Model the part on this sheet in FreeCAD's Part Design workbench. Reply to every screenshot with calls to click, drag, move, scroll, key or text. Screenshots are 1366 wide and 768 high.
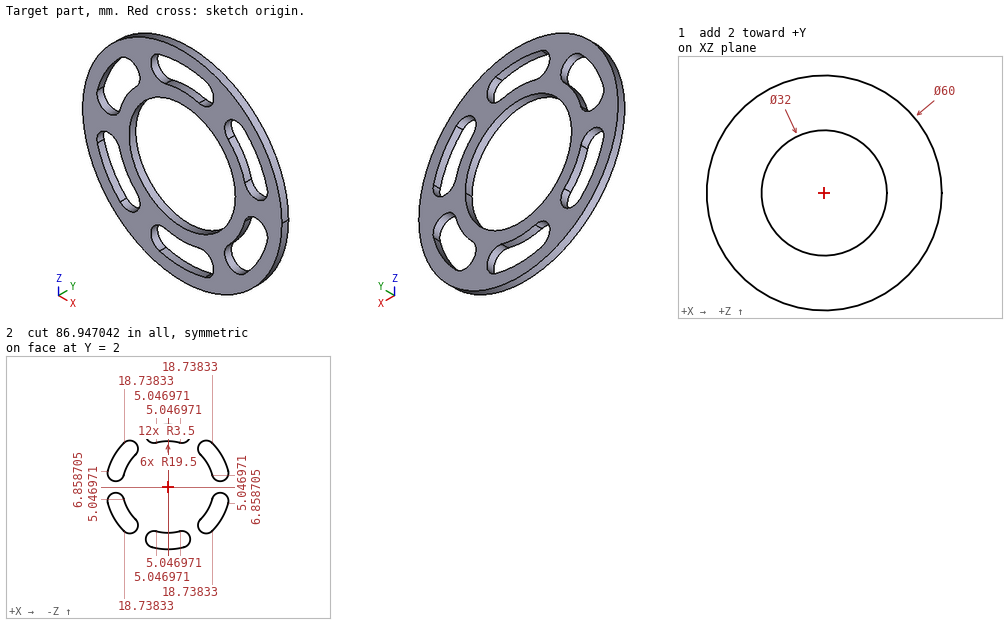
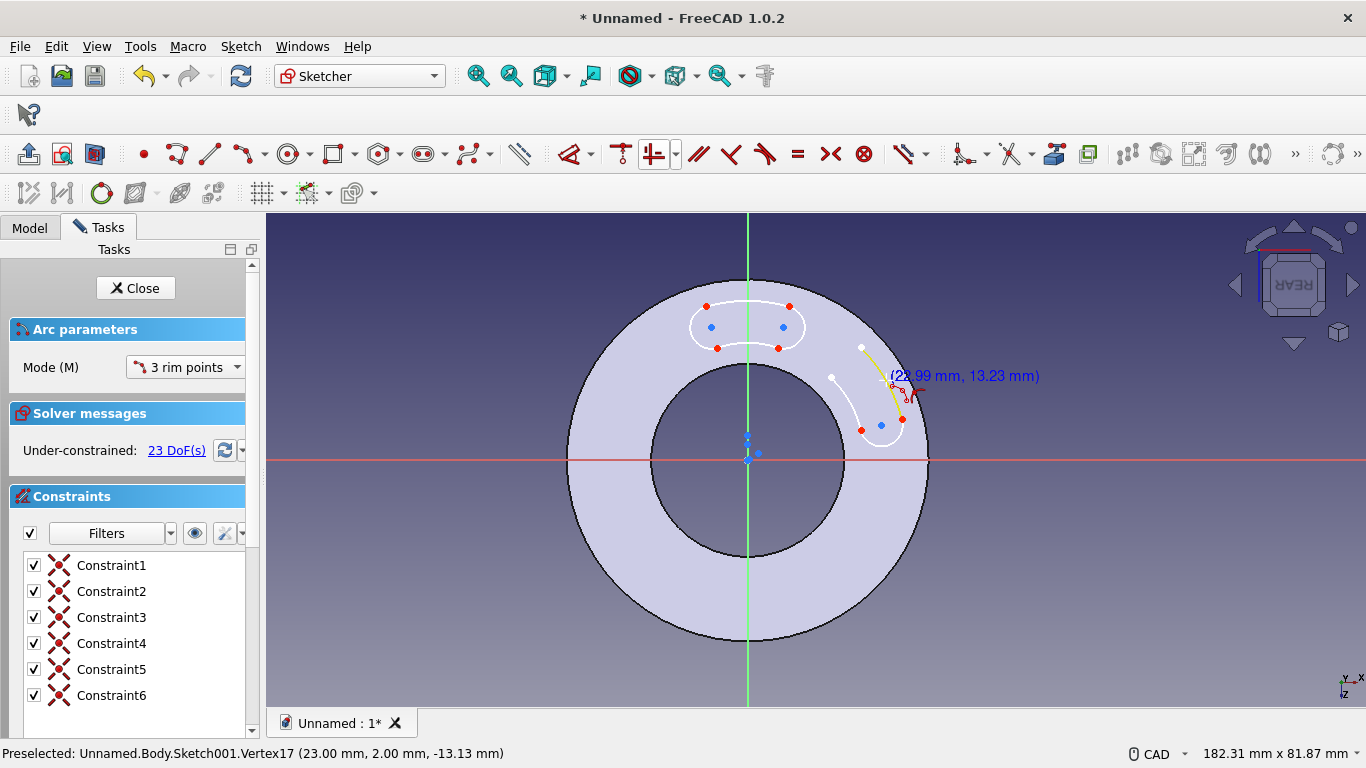
click(861, 348)
click(831, 378)
click(831, 347)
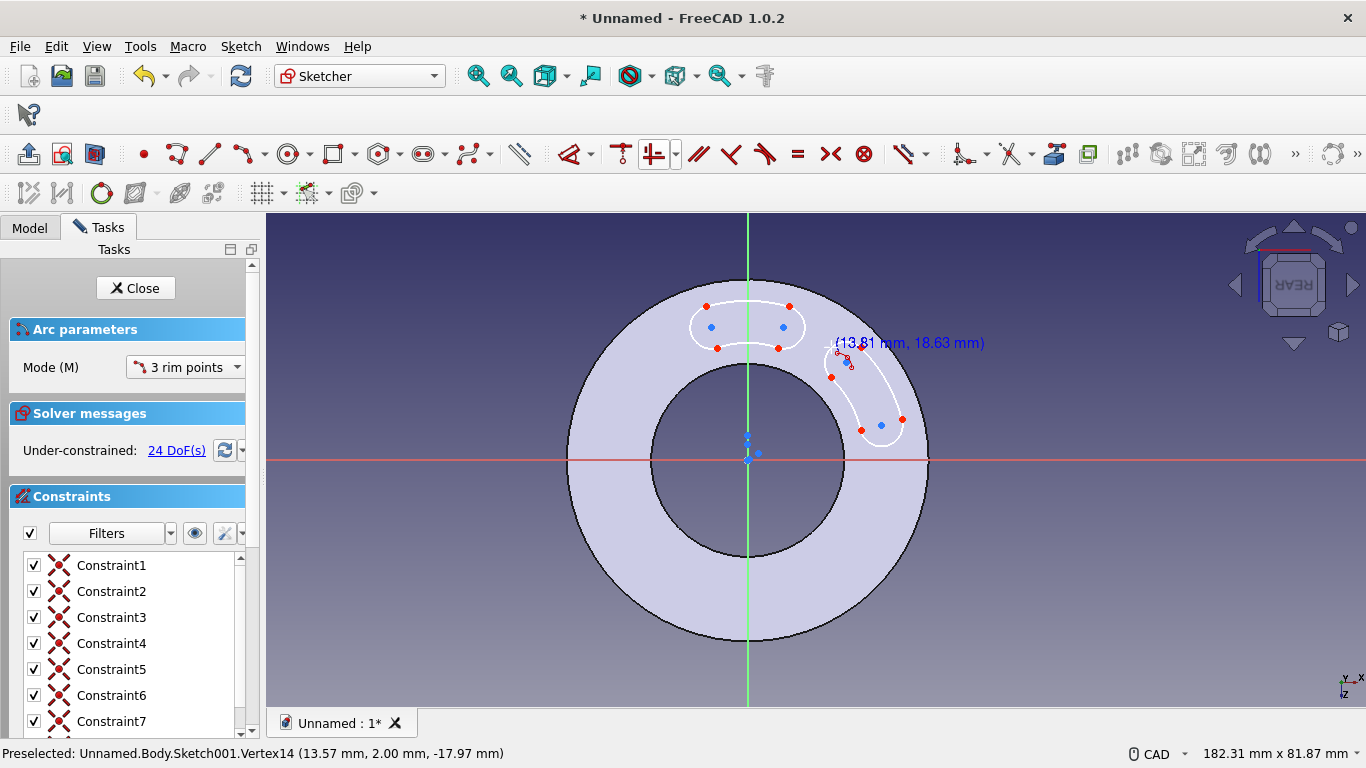
click(831, 544)
click(861, 573)
click(831, 573)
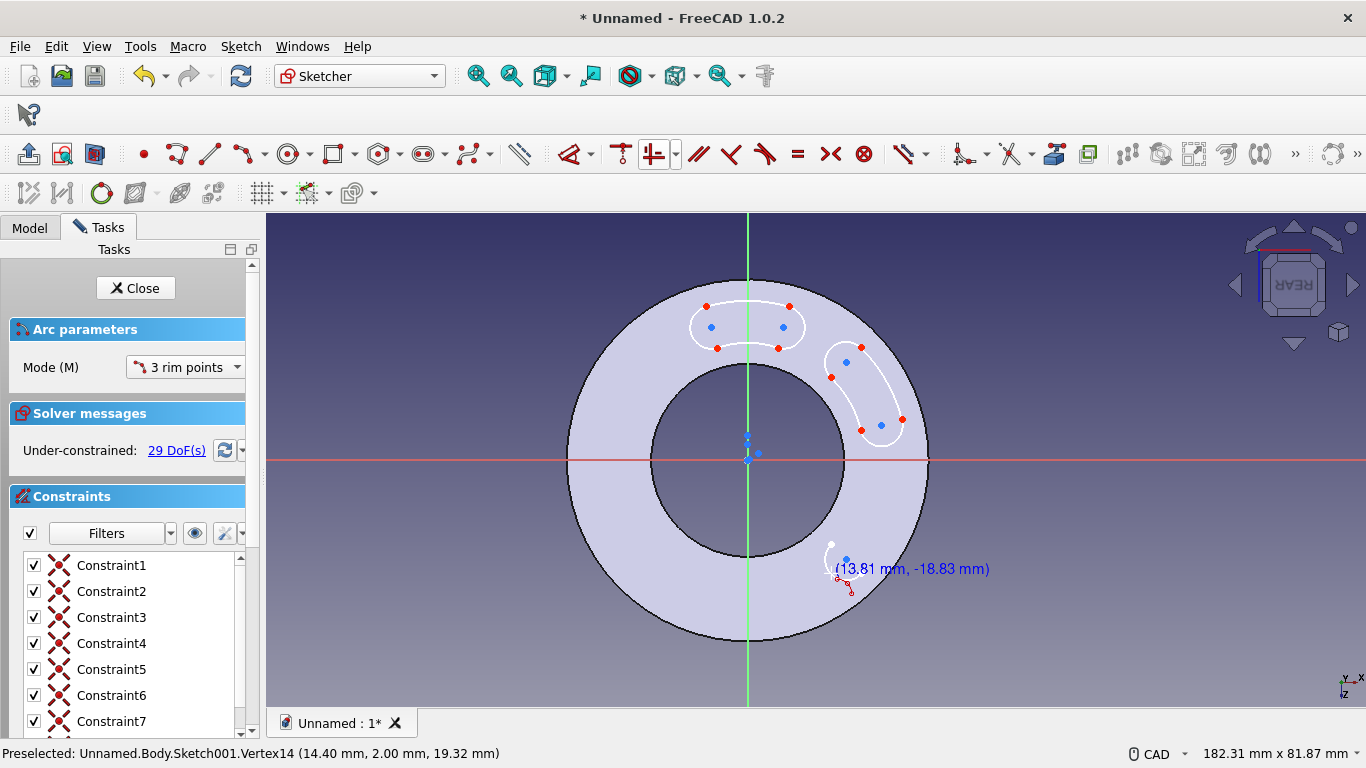
click(861, 574)
click(902, 502)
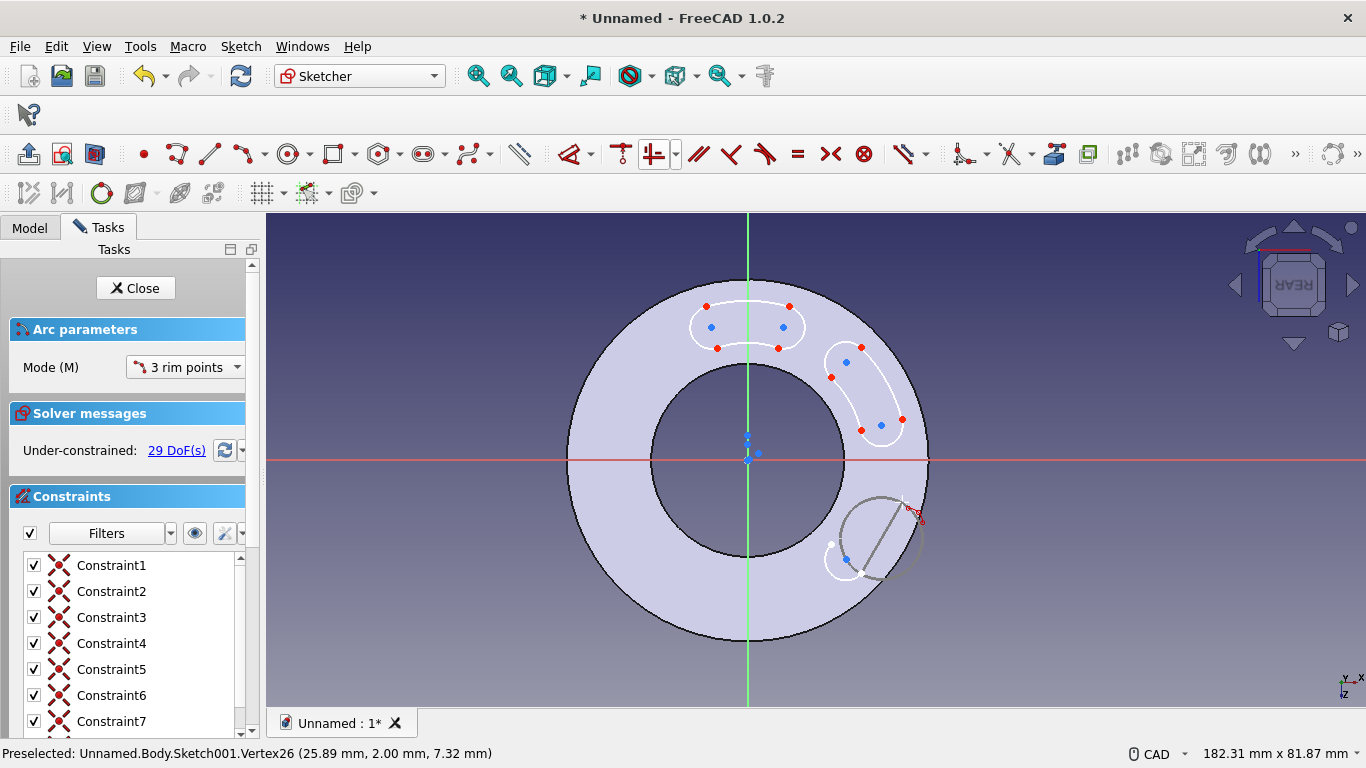
scroll(886, 540, up, 6)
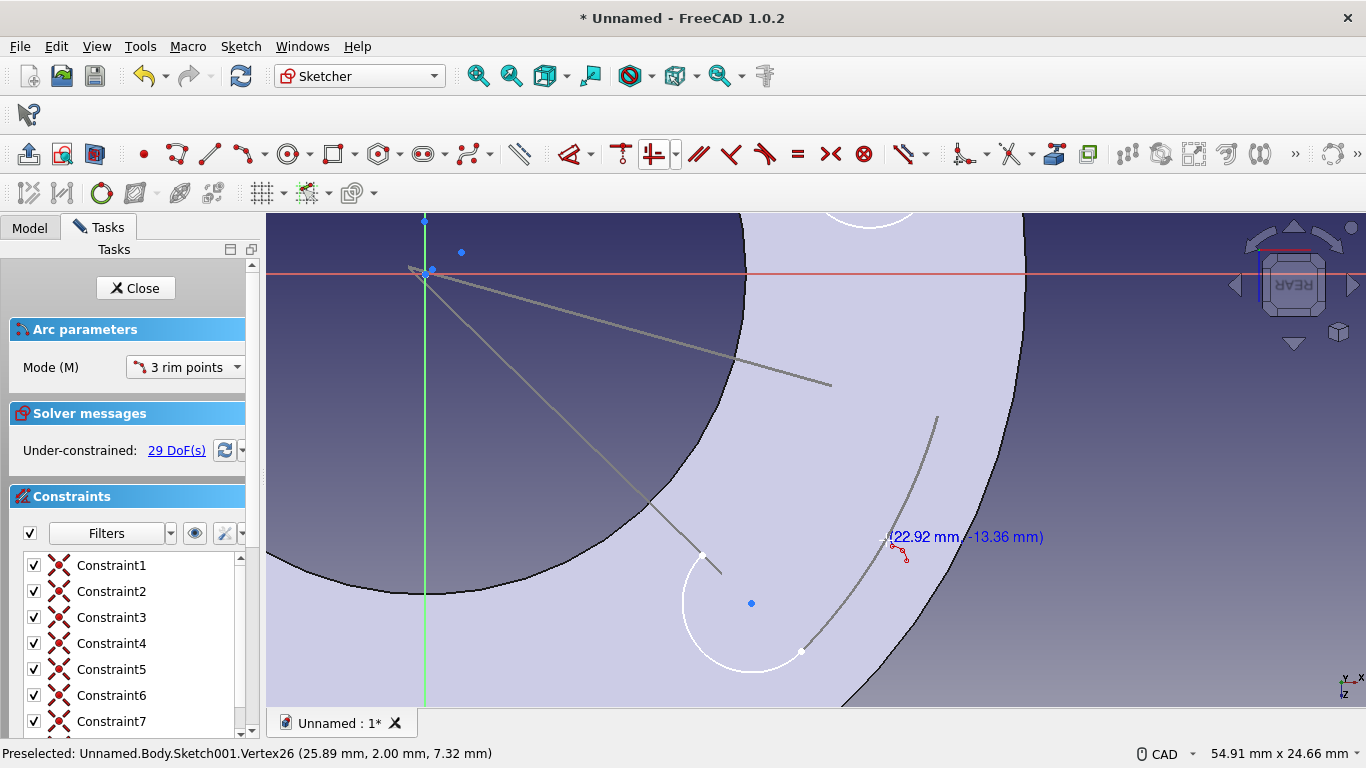
click(885, 540)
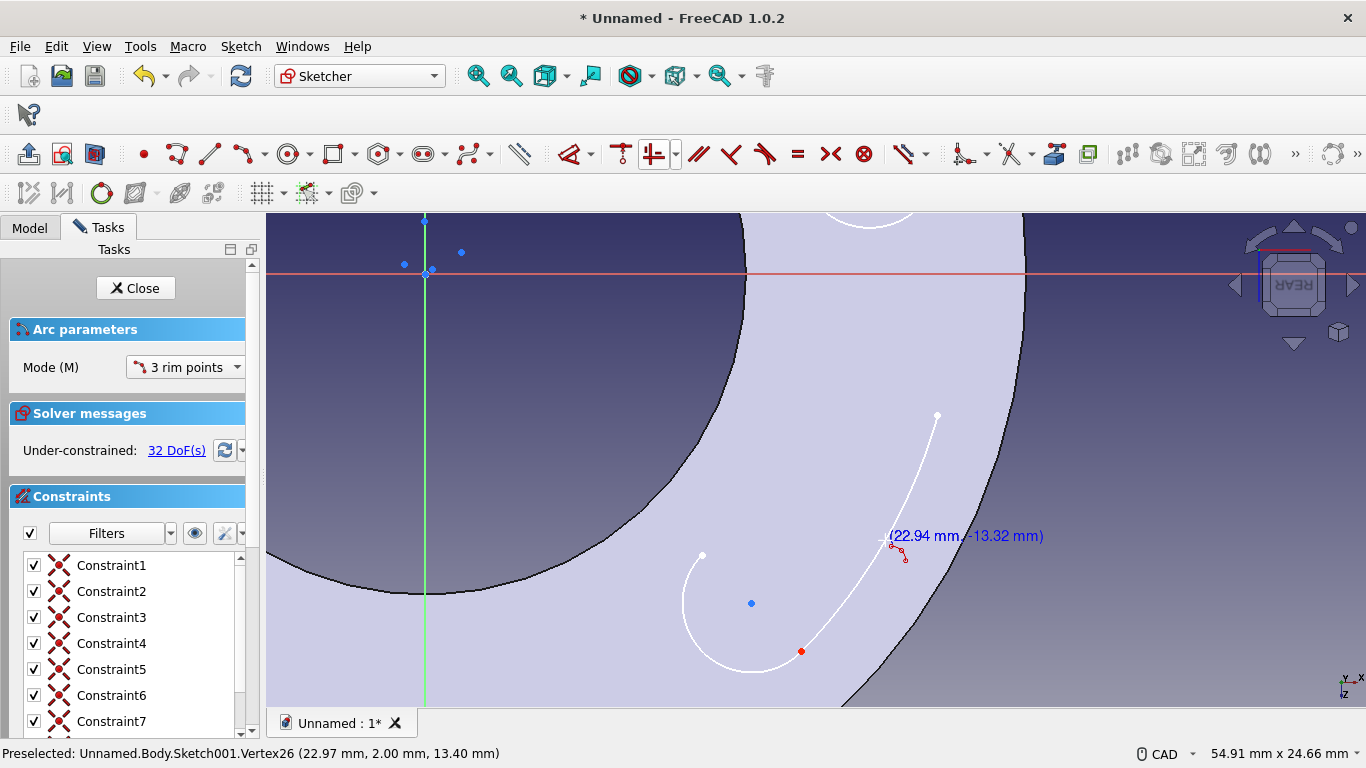
scroll(886, 540, down, 6)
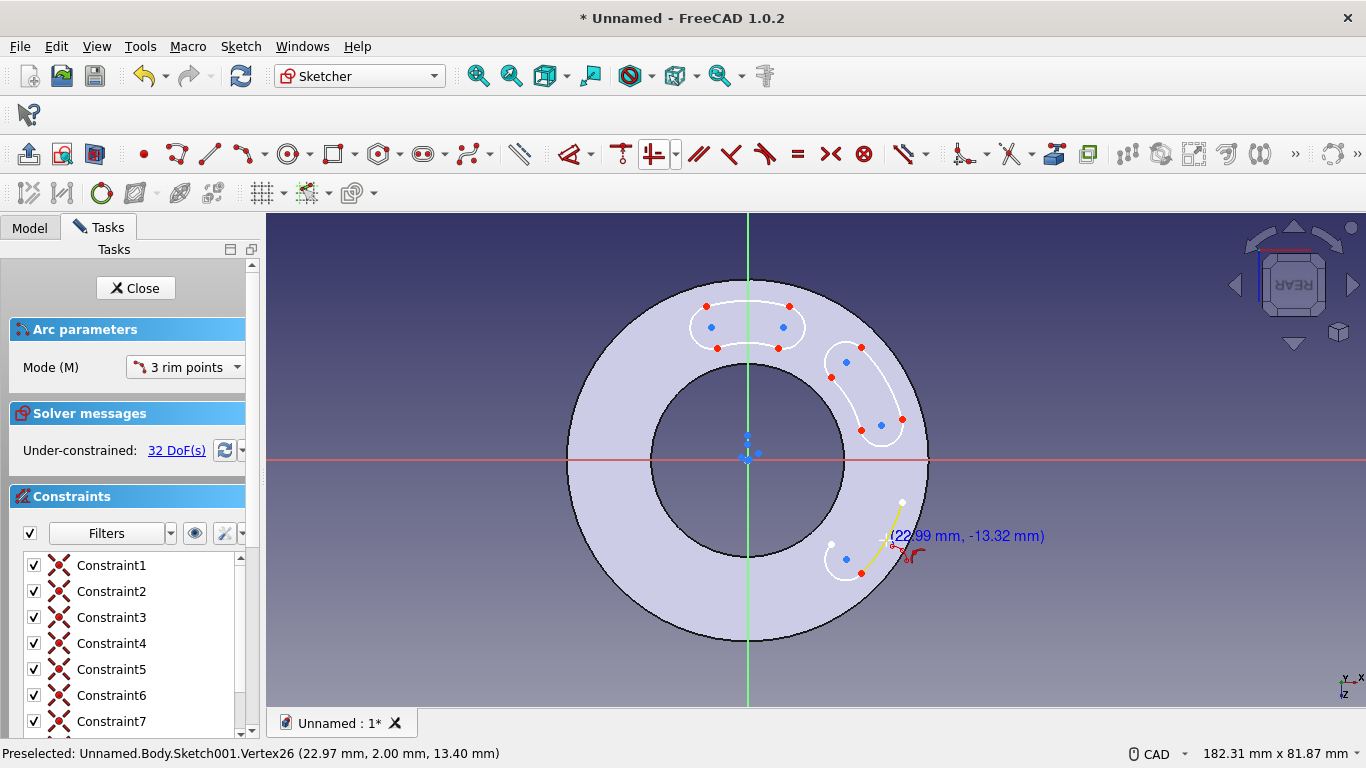
click(902, 503)
click(861, 491)
click(893, 479)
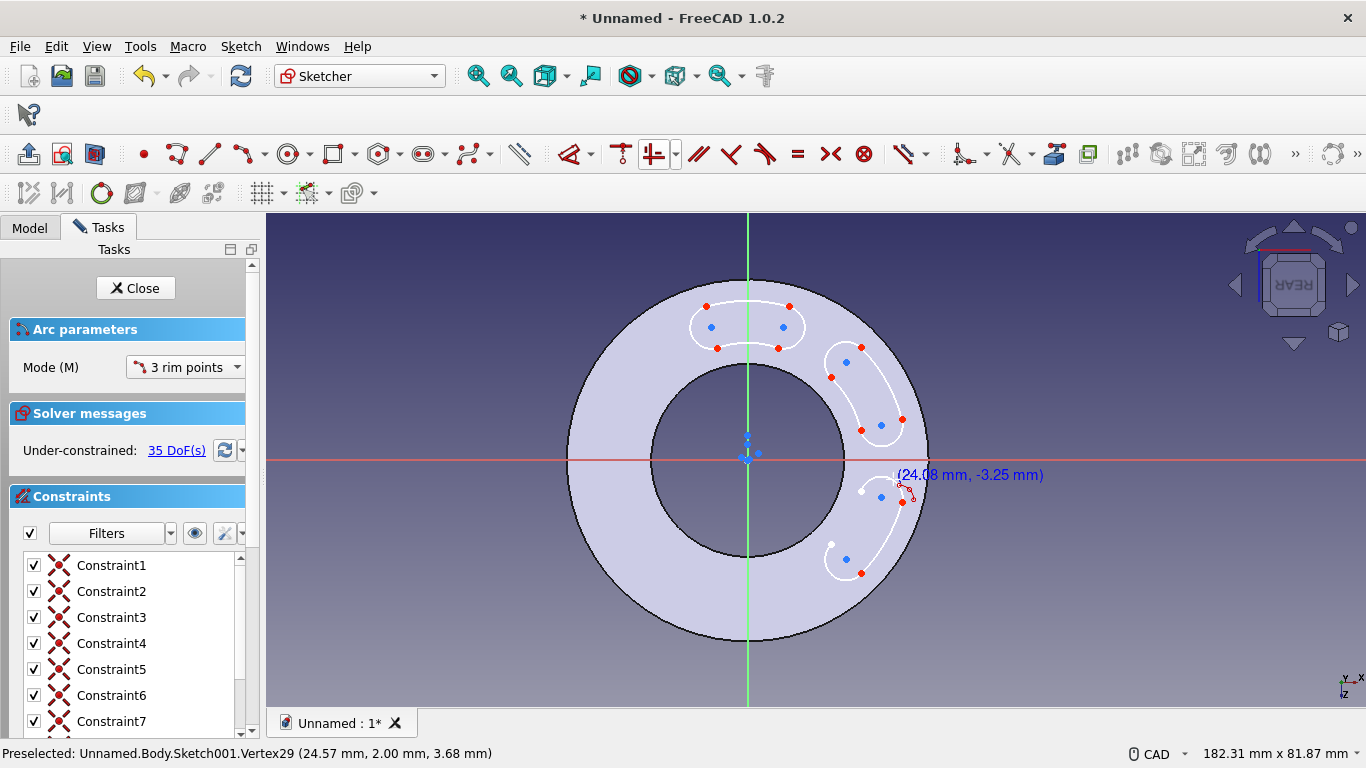
click(861, 492)
click(831, 545)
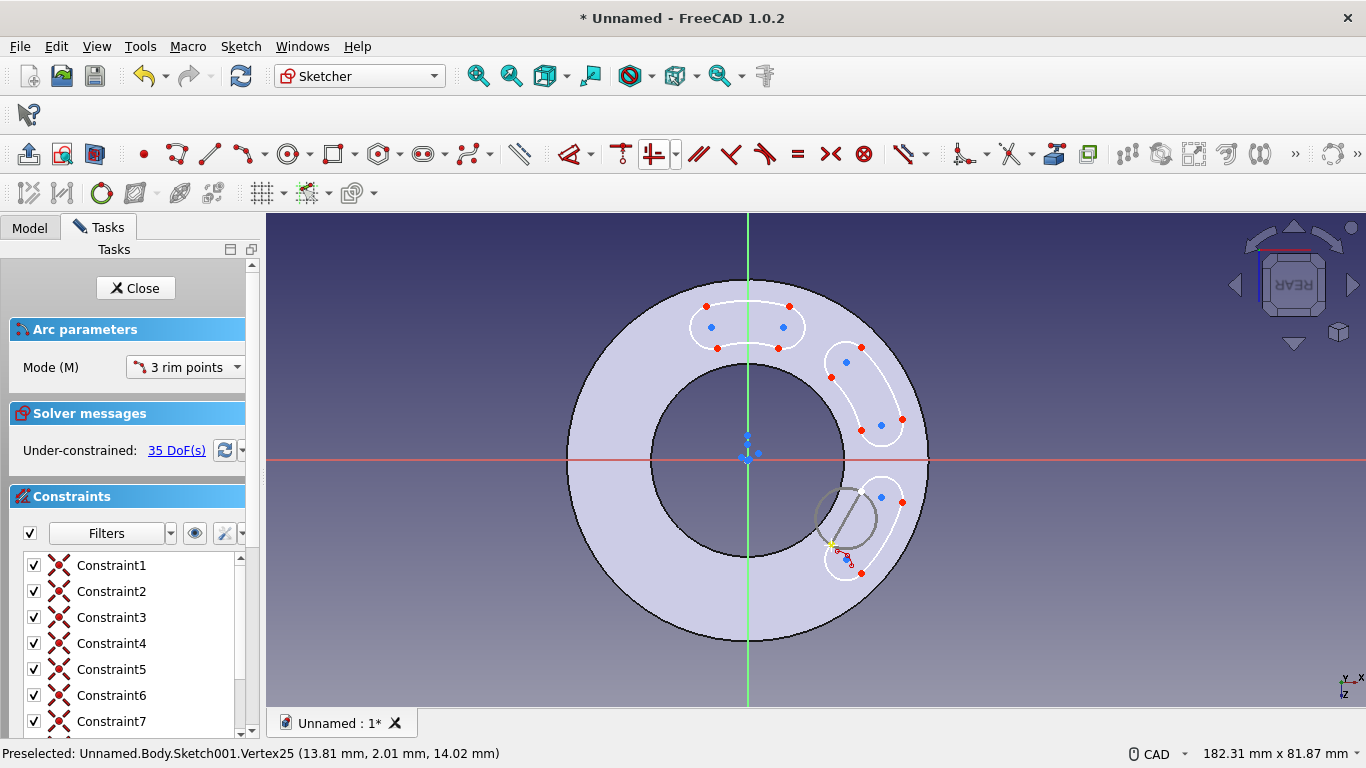
scroll(850, 519, up, 7)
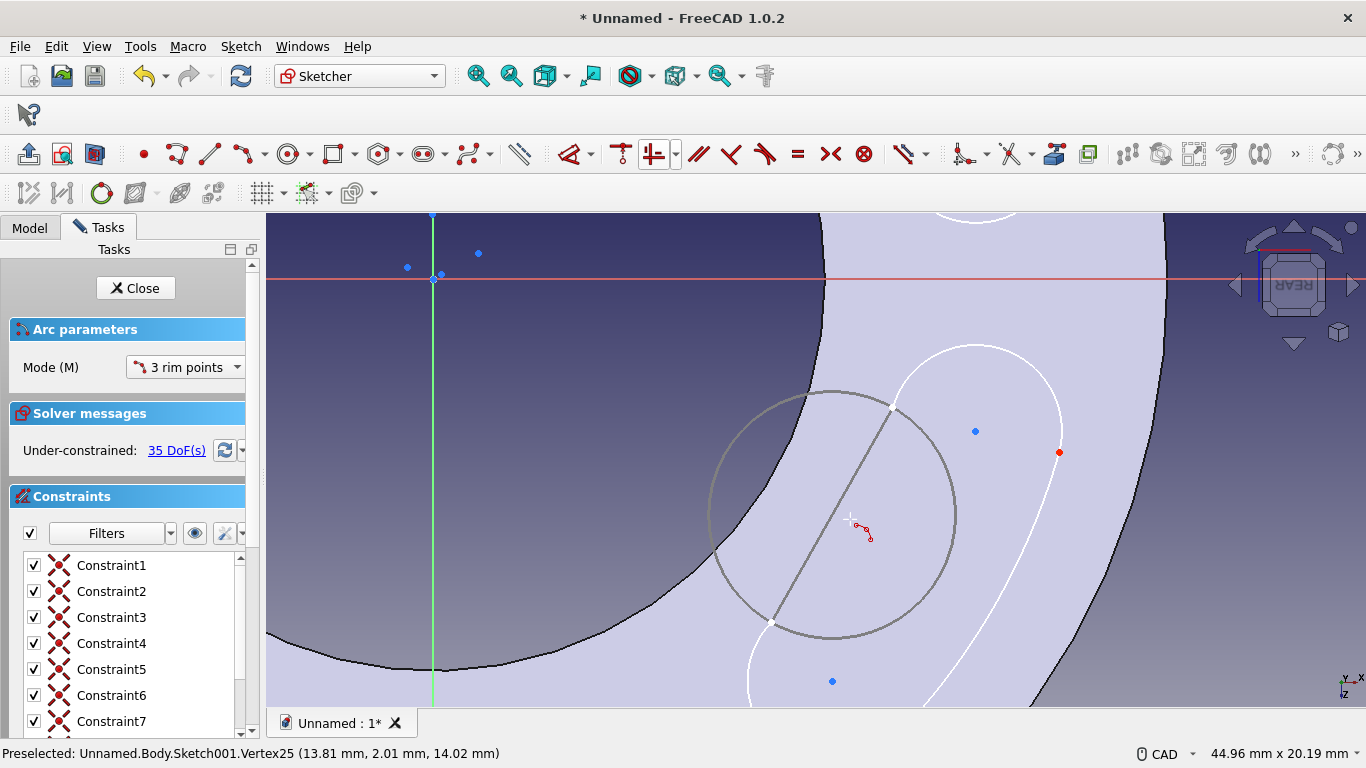
click(847, 518)